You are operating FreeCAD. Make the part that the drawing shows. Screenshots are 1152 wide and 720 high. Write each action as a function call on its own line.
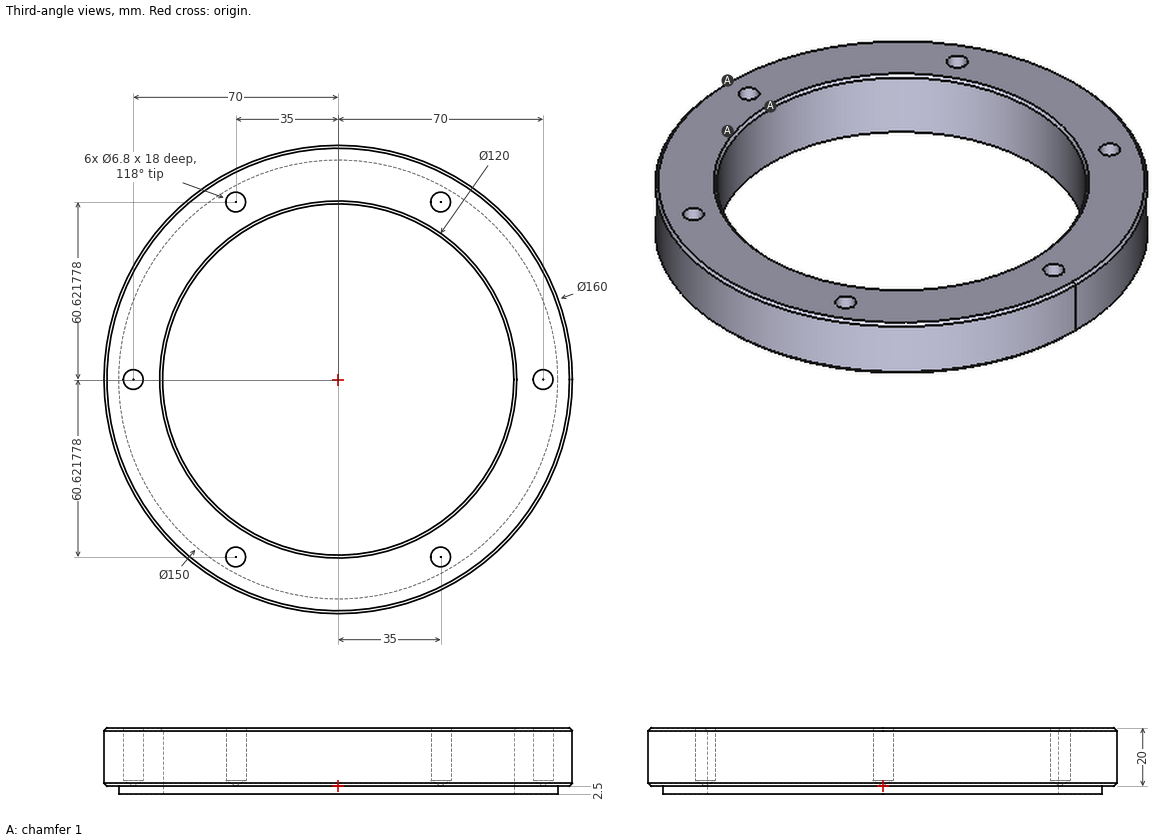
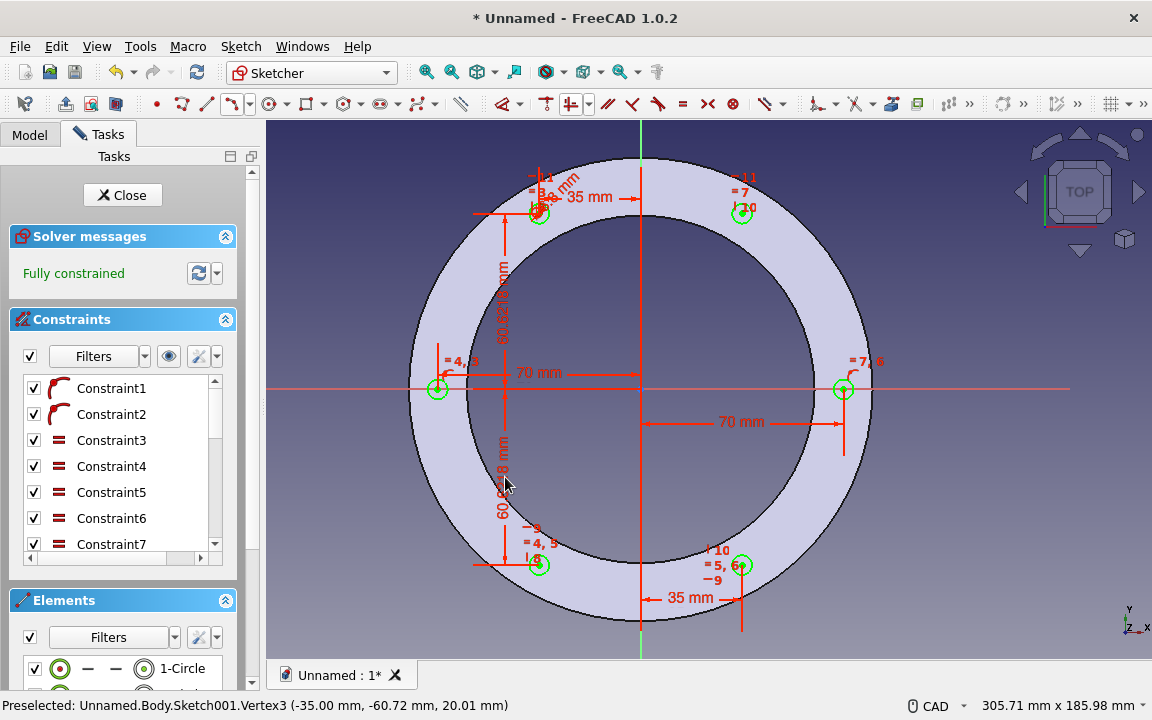
click(123, 195)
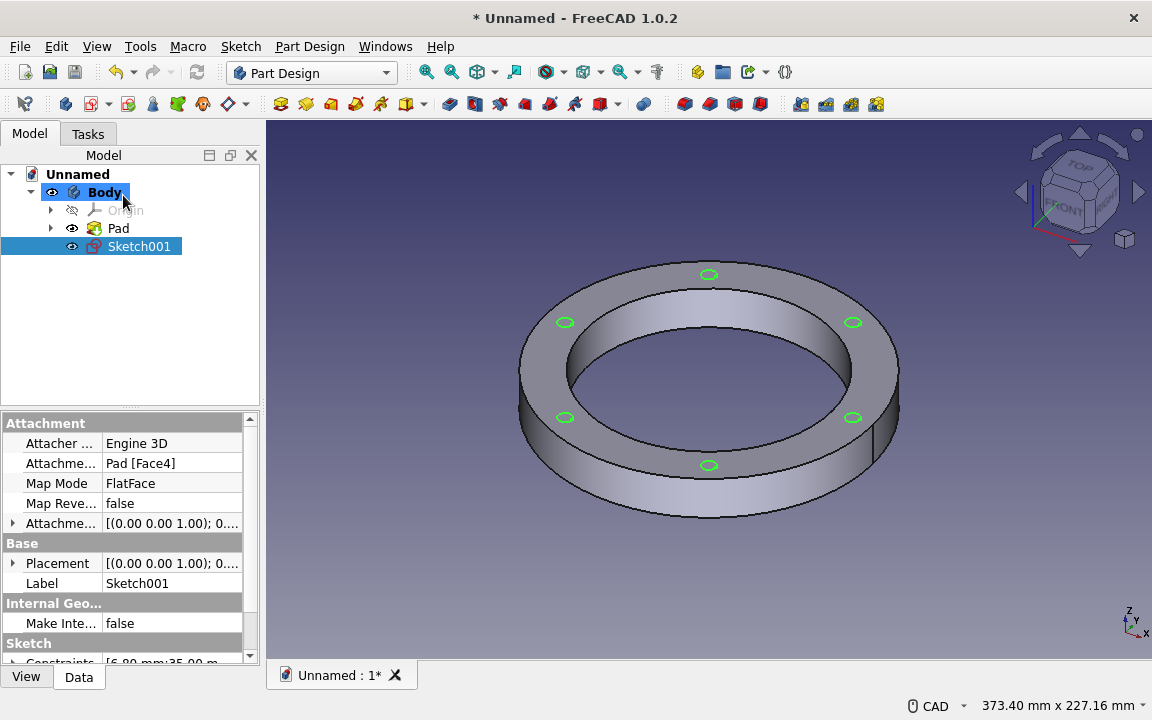
click(475, 104)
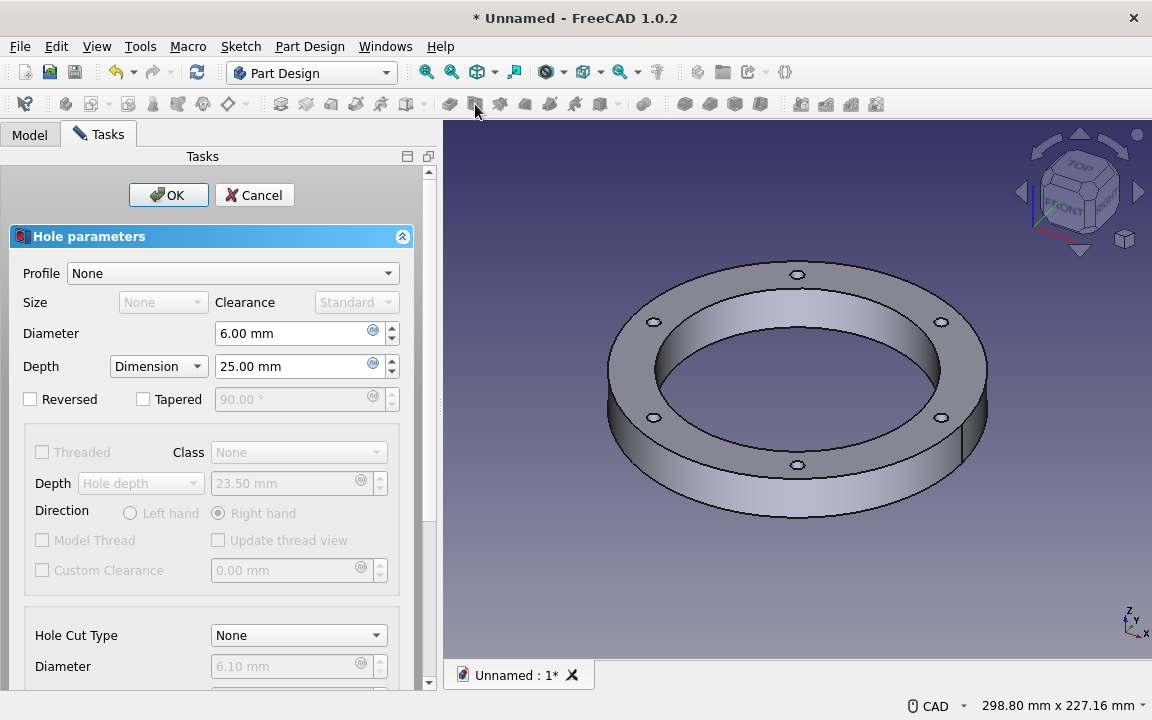
triple_click(300, 334)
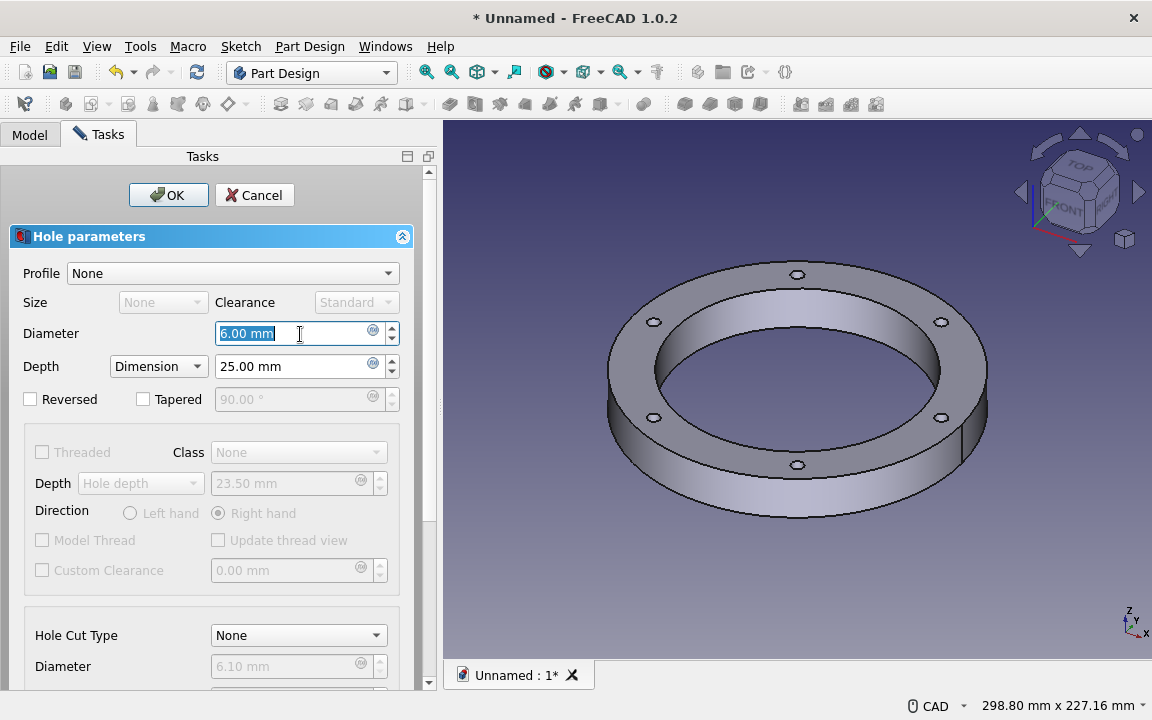
text(6.8)
key(Tab)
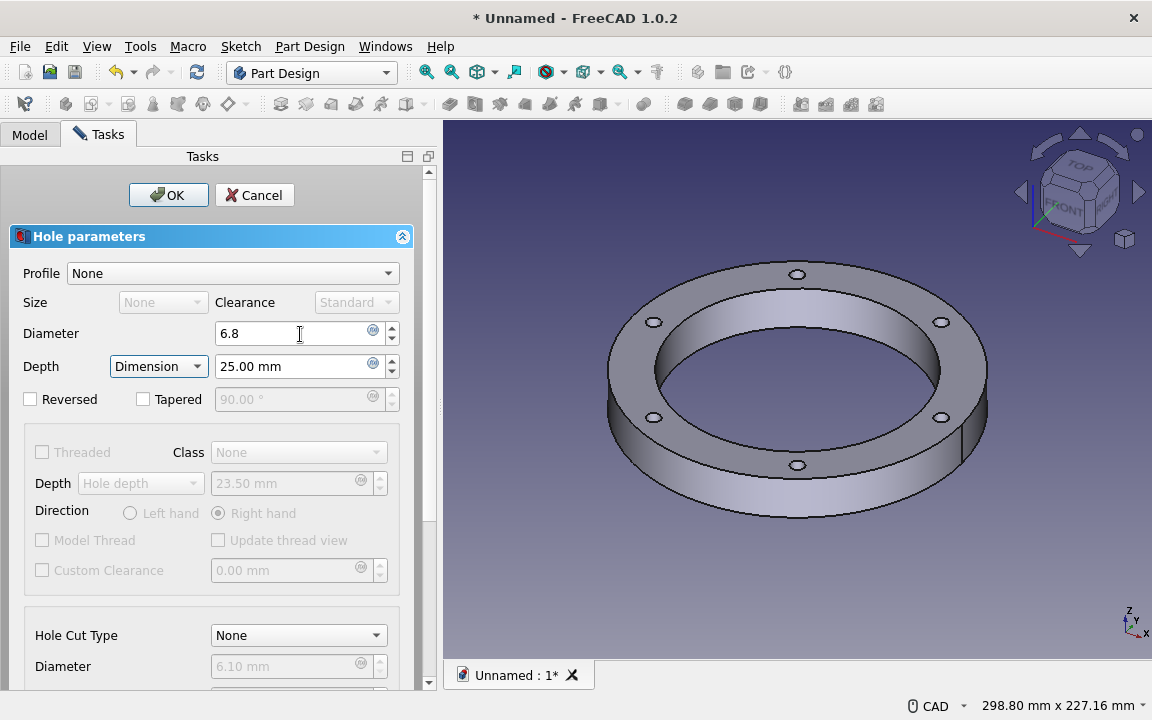
triple_click(300, 366)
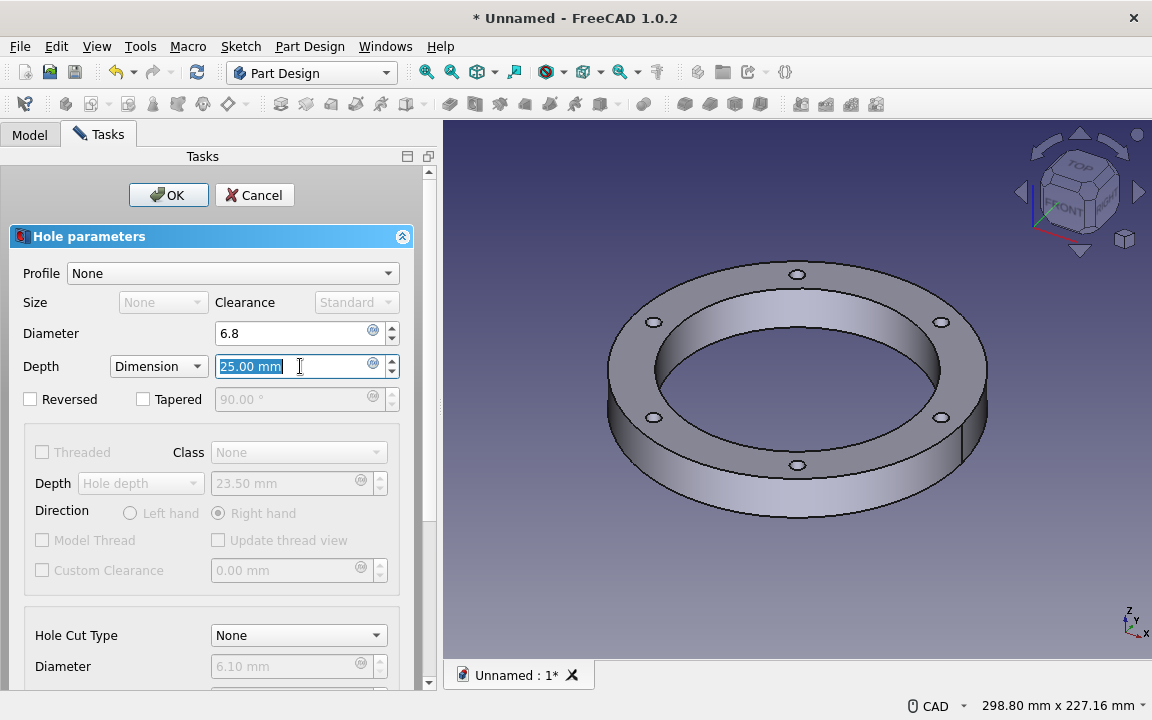
text(18)
key(Tab)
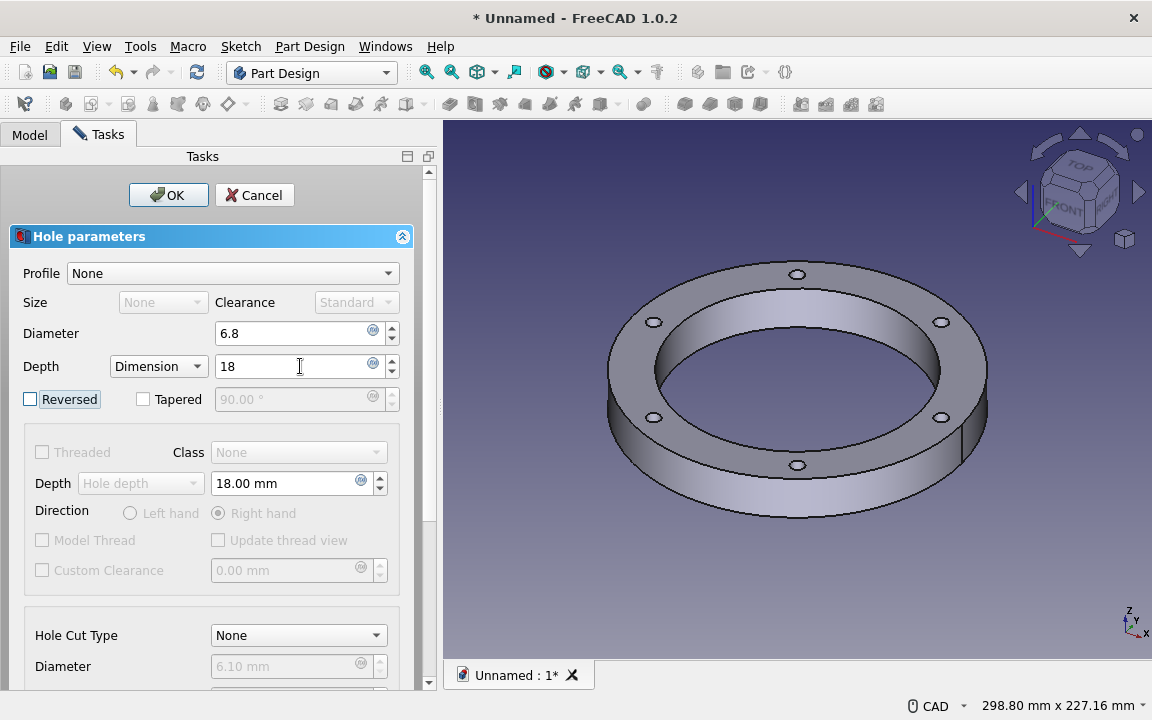
click(169, 195)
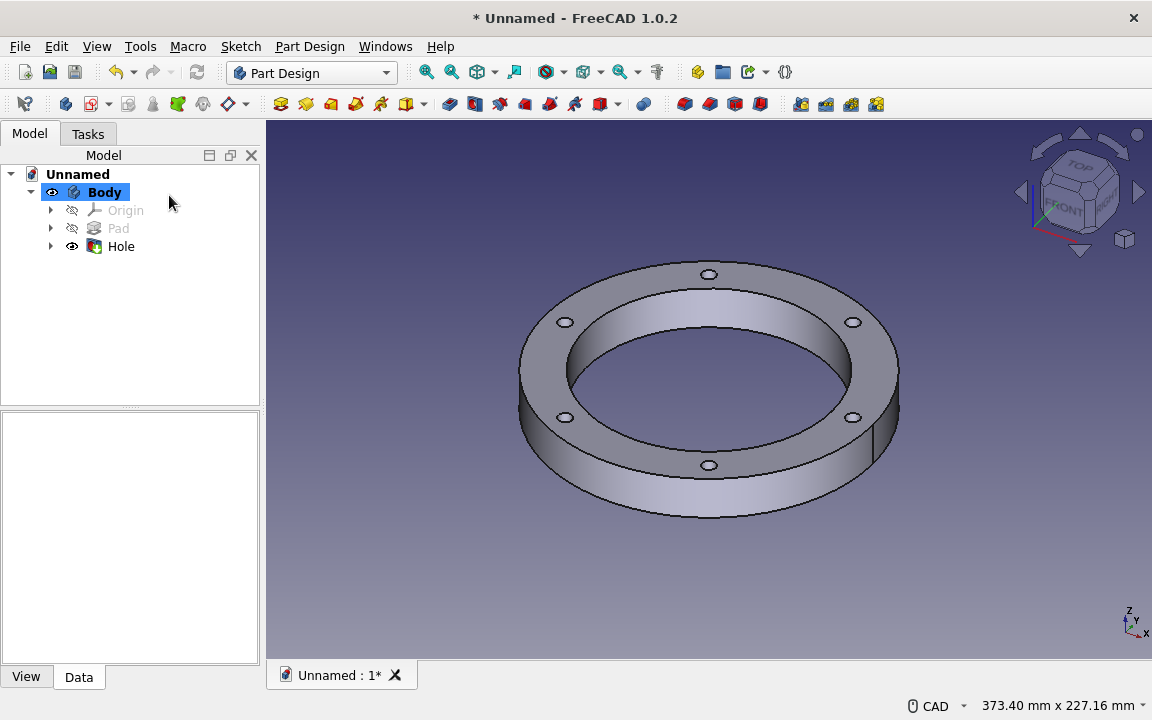
click(520, 380)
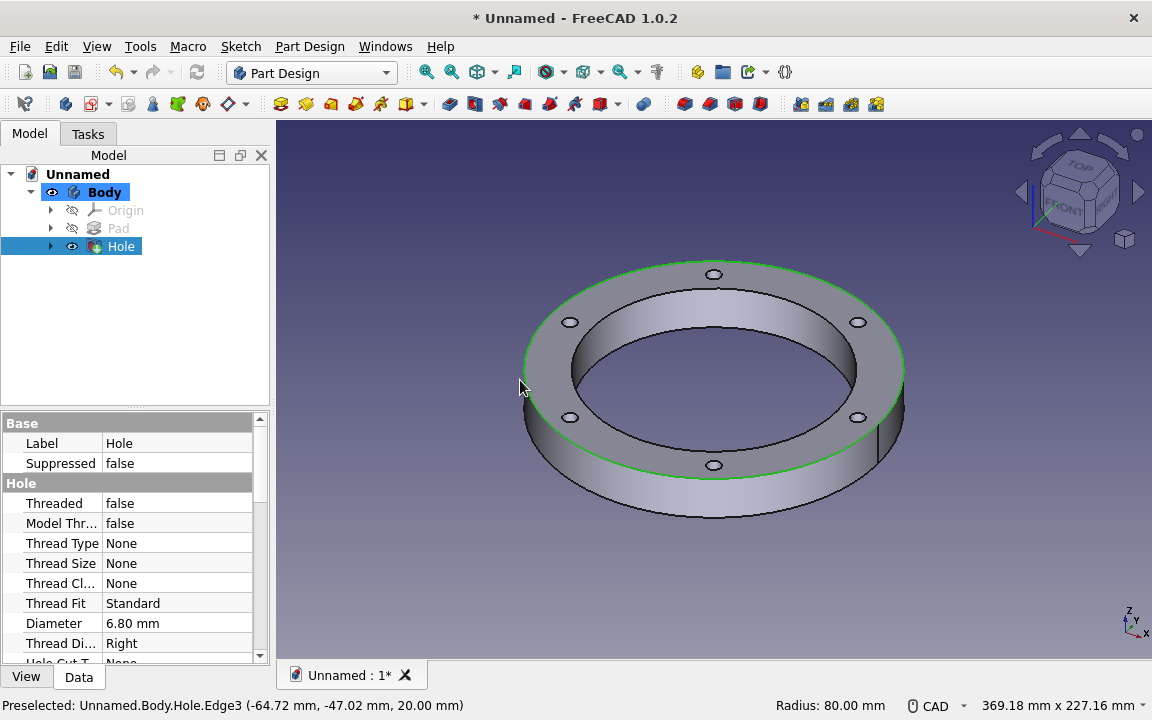
click(591, 328, ctrl)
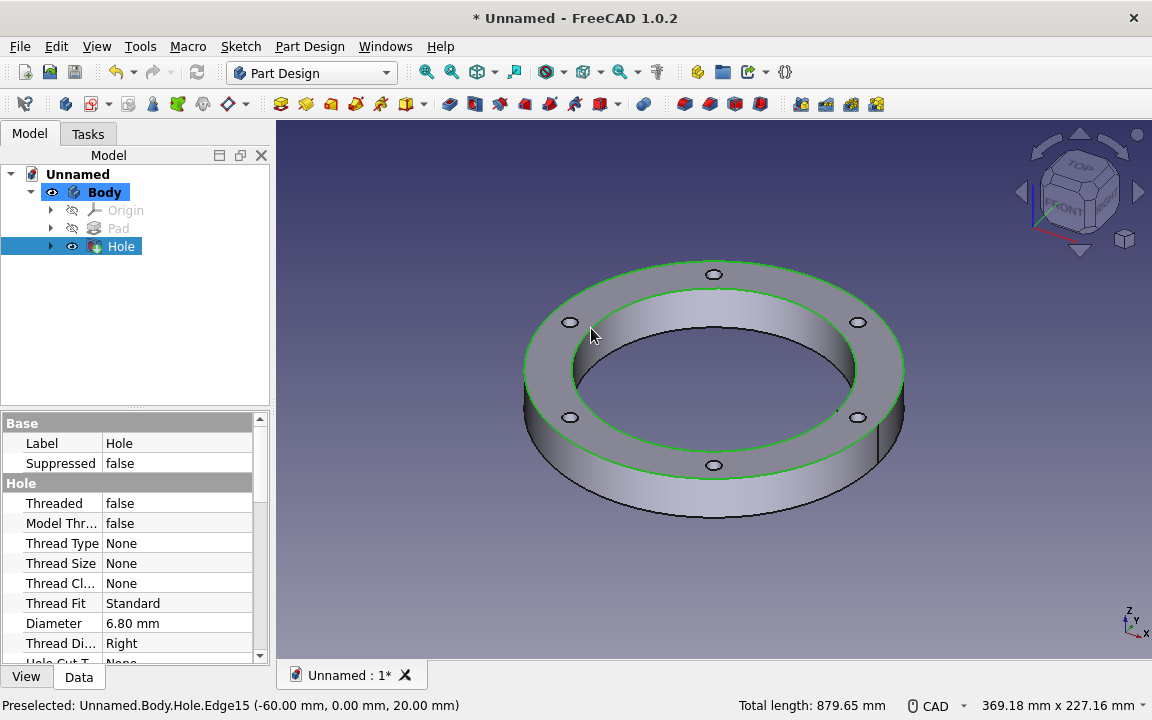
key(0)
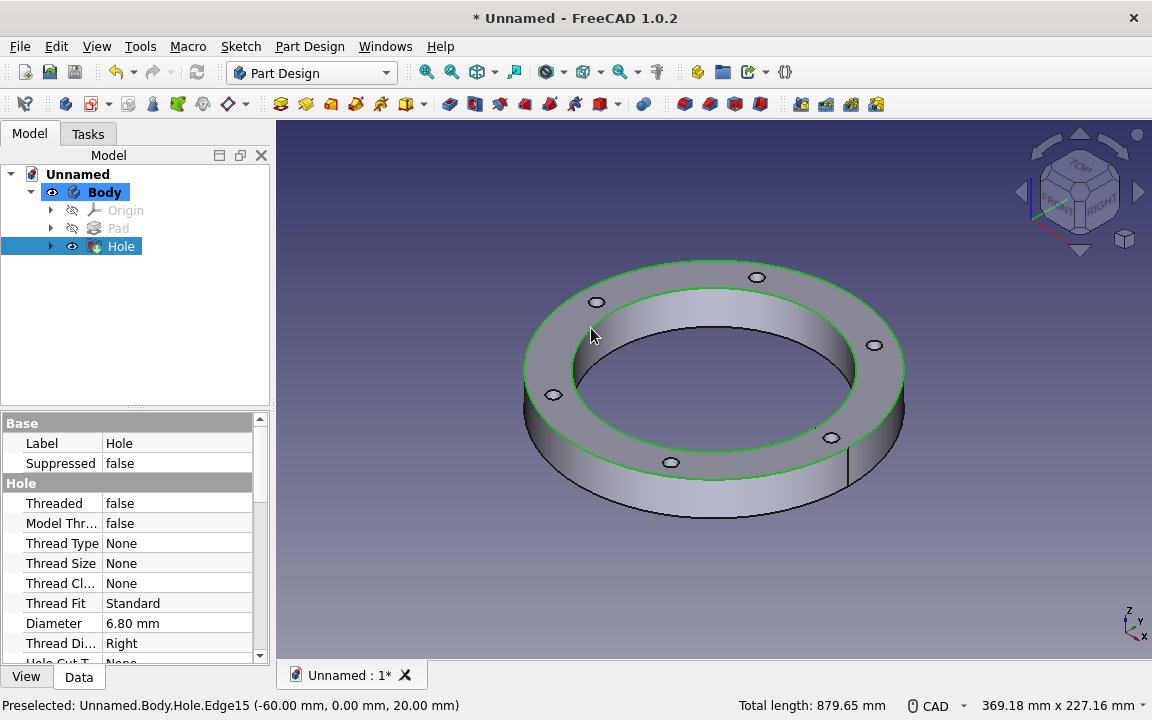
key(2)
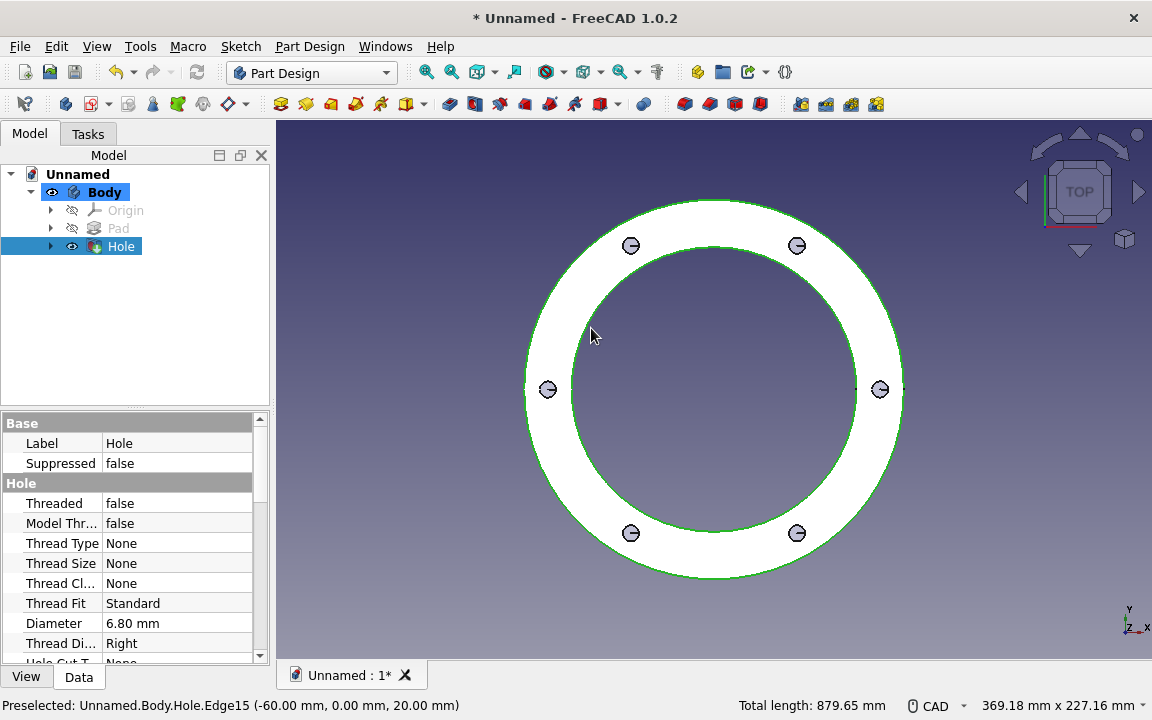
key(1)